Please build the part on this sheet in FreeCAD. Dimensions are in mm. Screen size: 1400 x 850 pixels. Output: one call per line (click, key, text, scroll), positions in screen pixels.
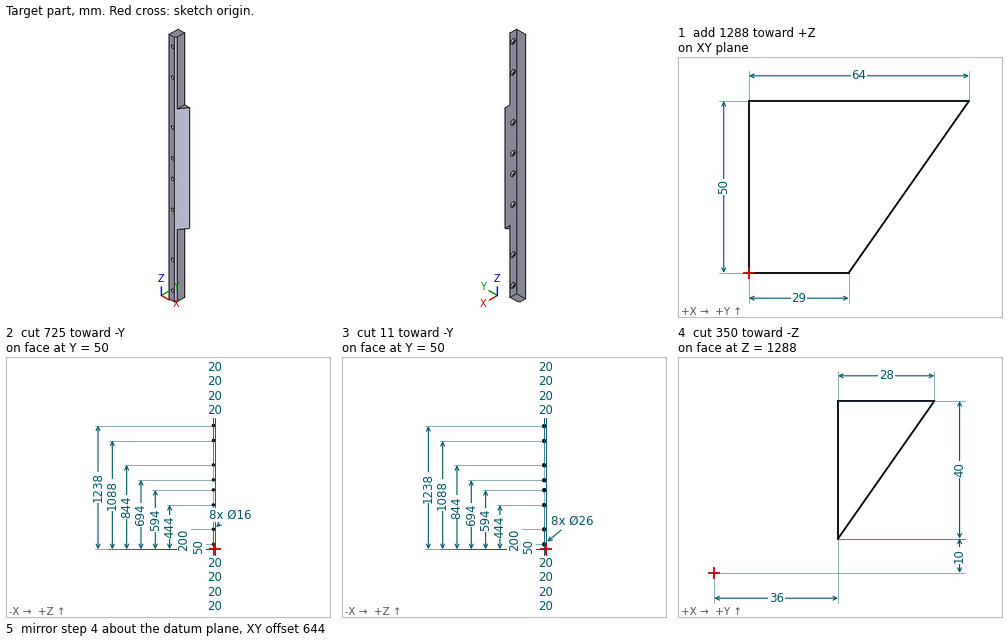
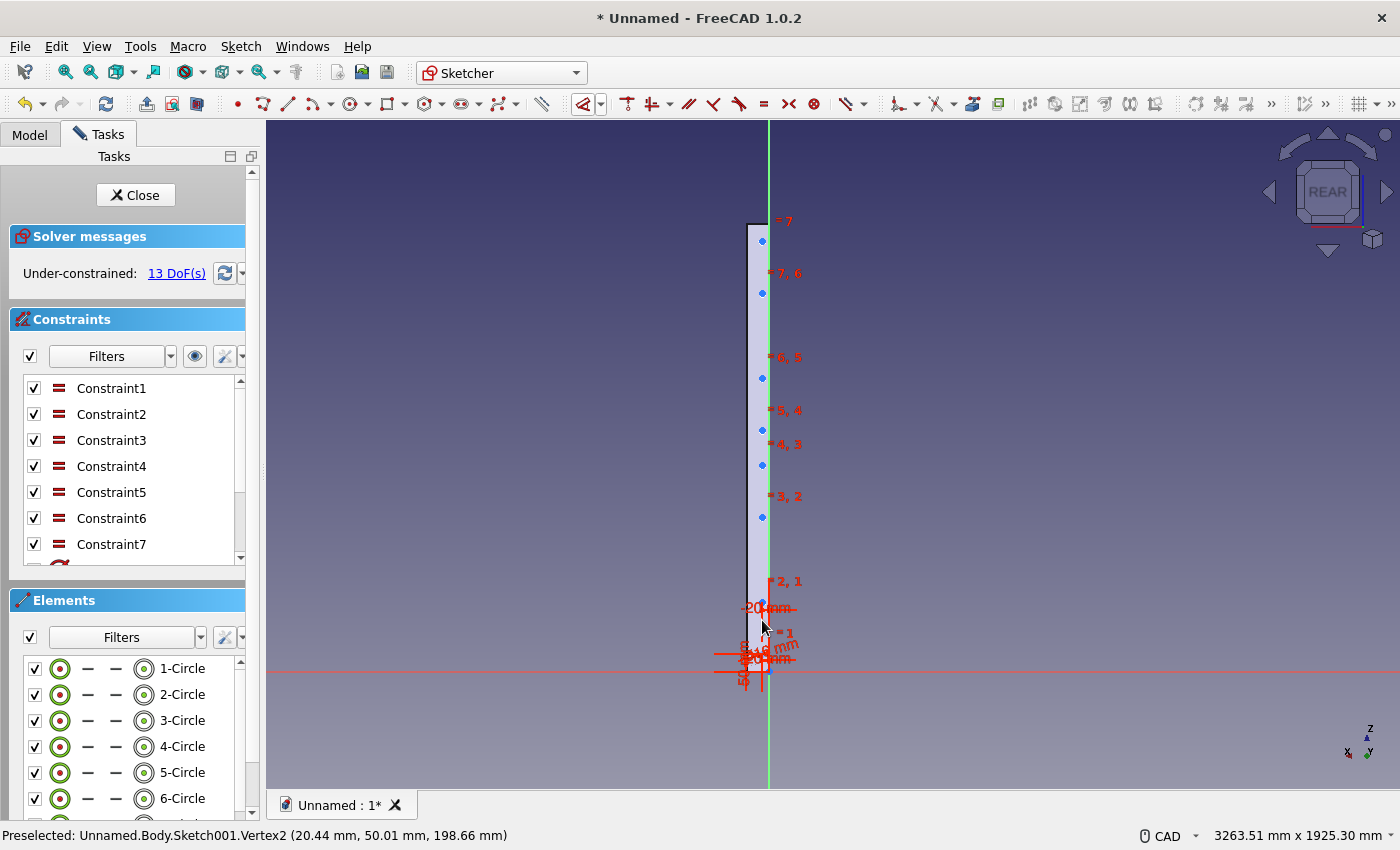
scroll(762, 518, up, 9)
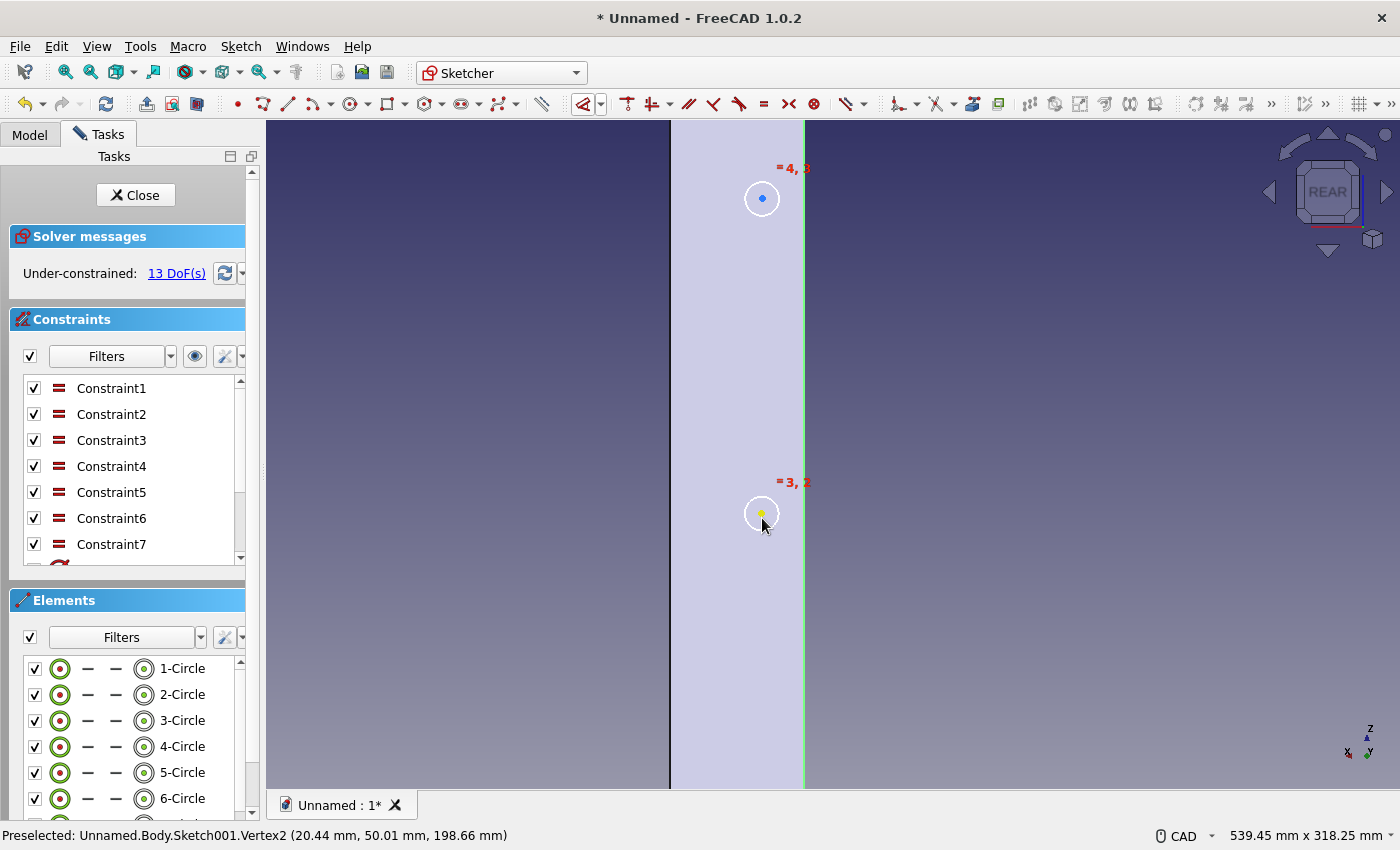
click(762, 514)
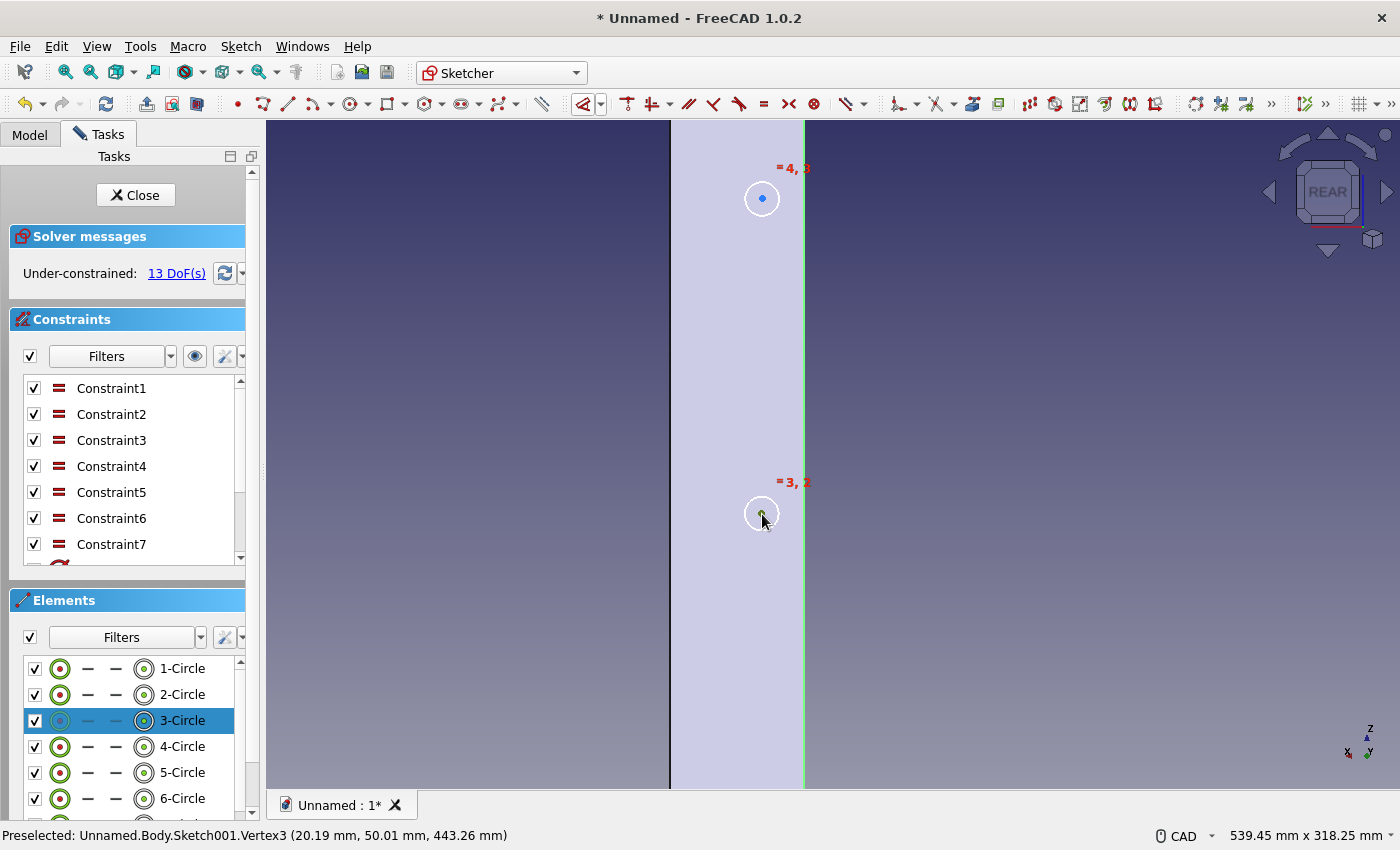
click(600, 104)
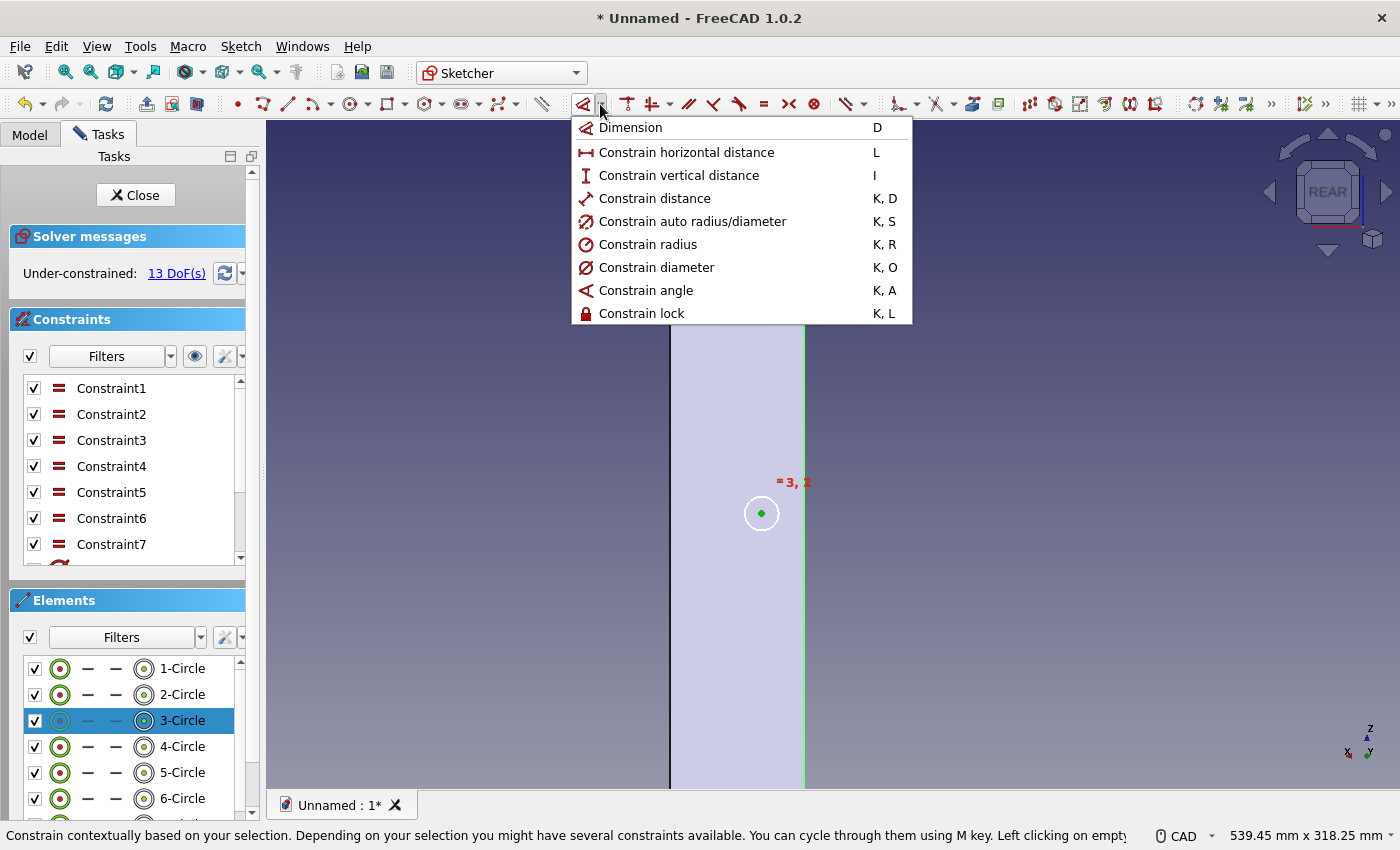
click(742, 152)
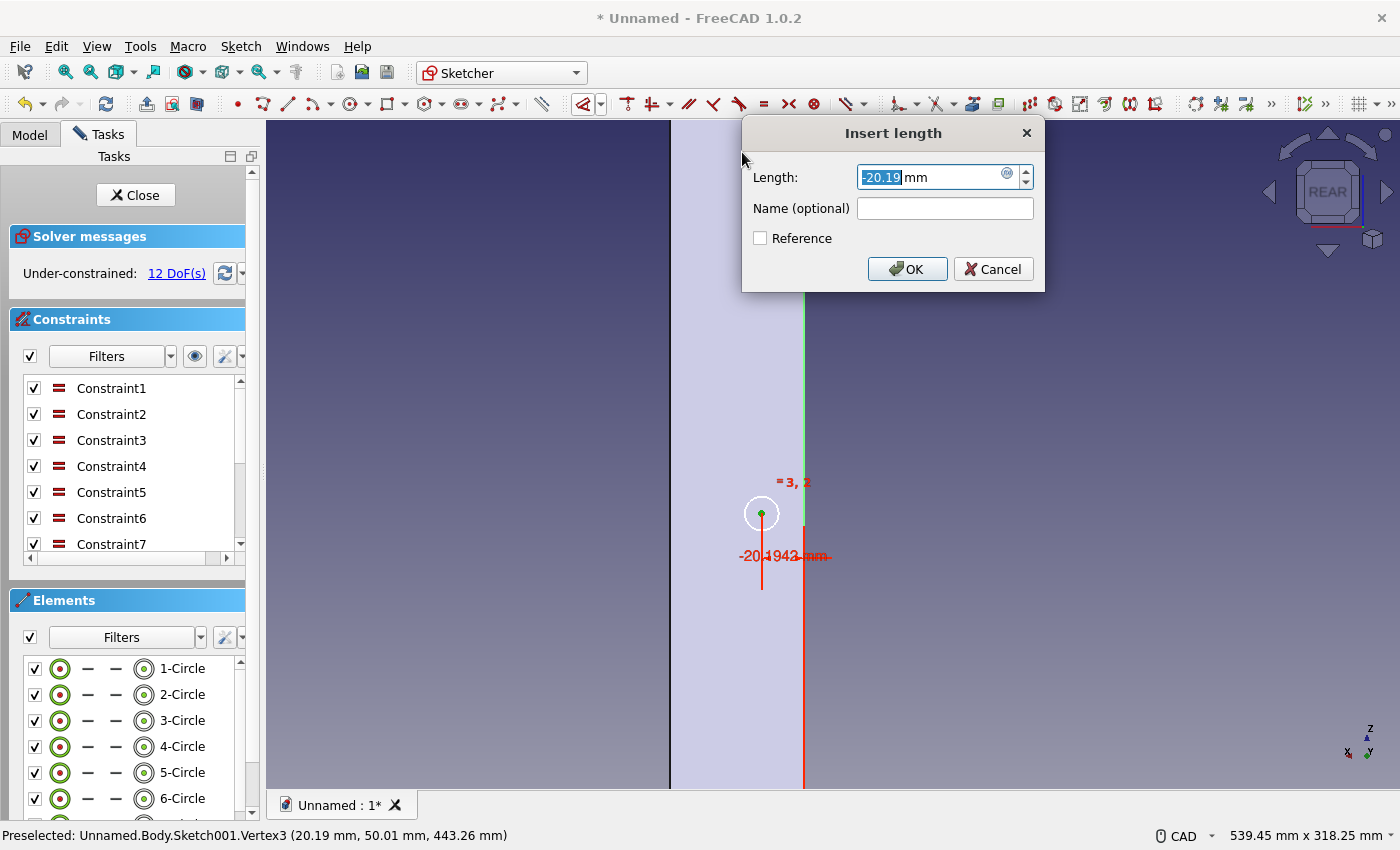
text(-20)
key(Return)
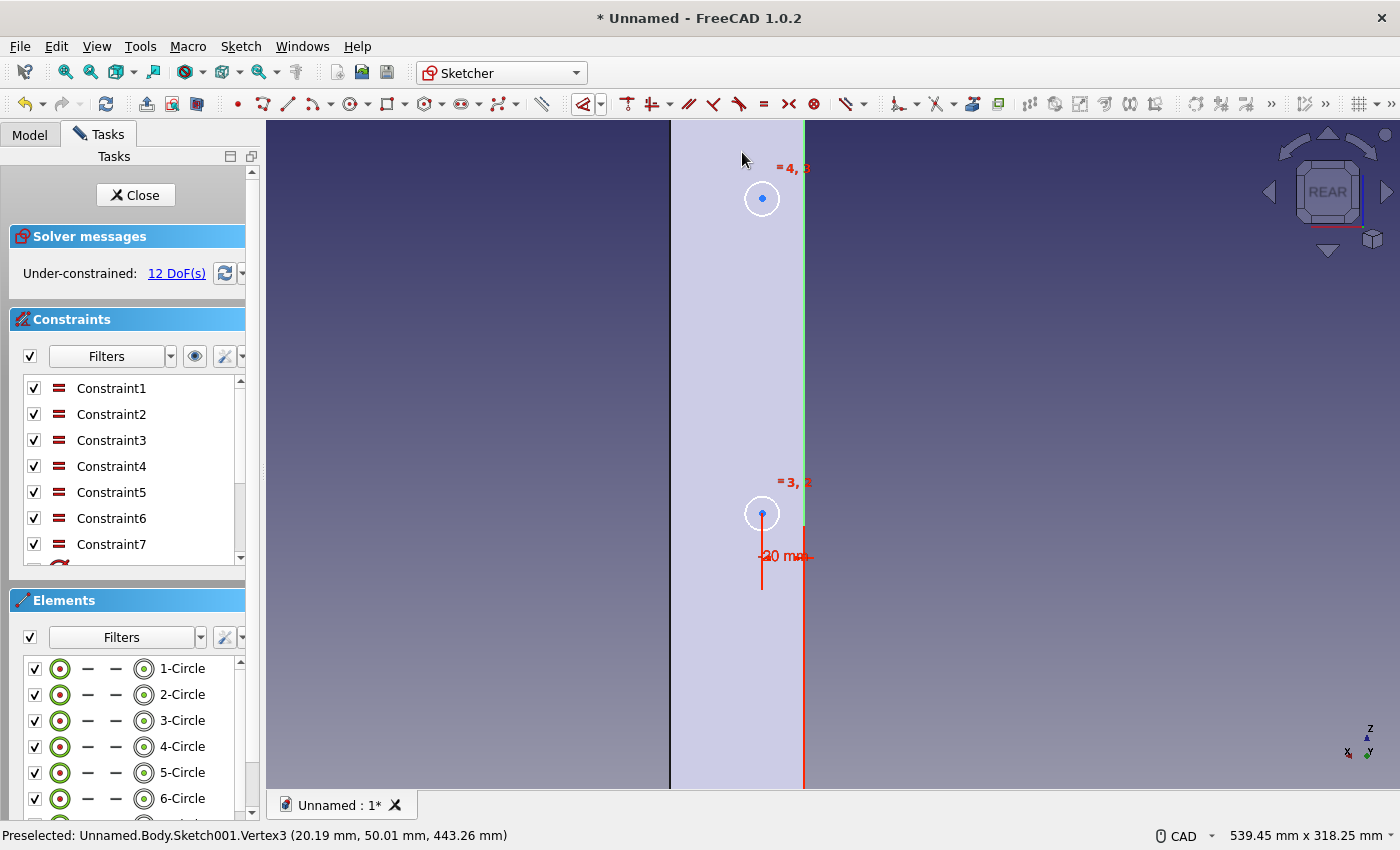
click(762, 199)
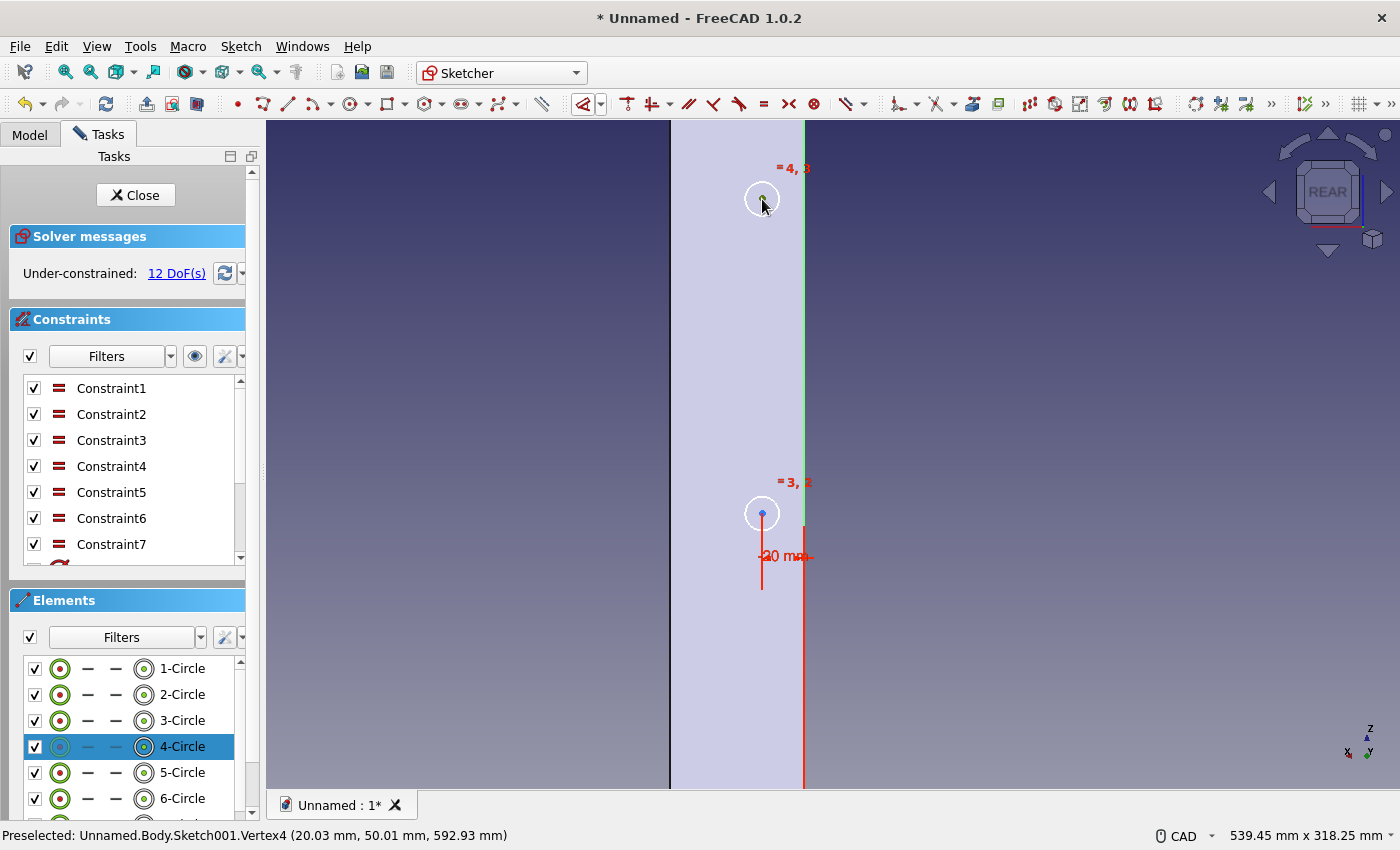
key(l)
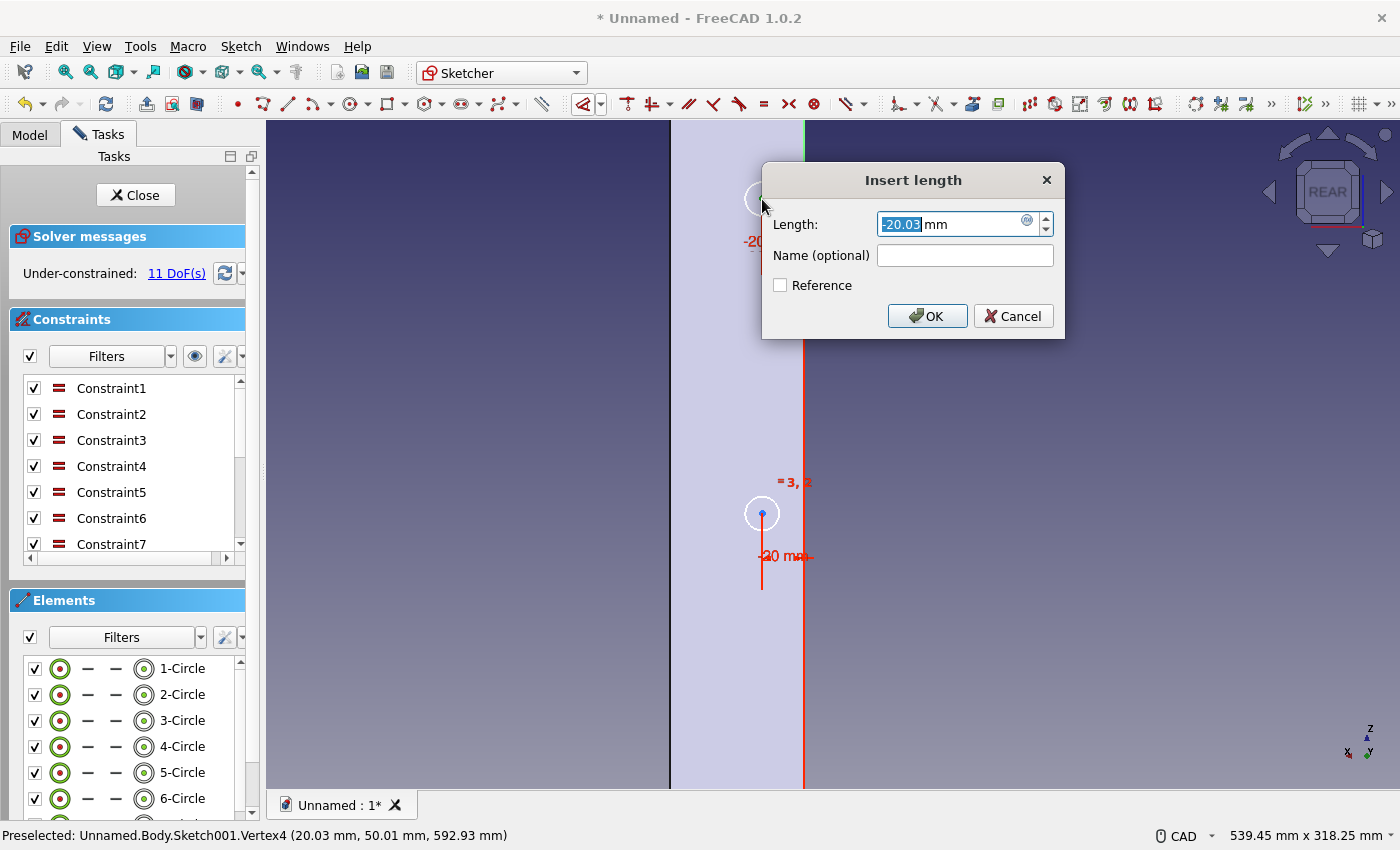
text(-20)
key(Return)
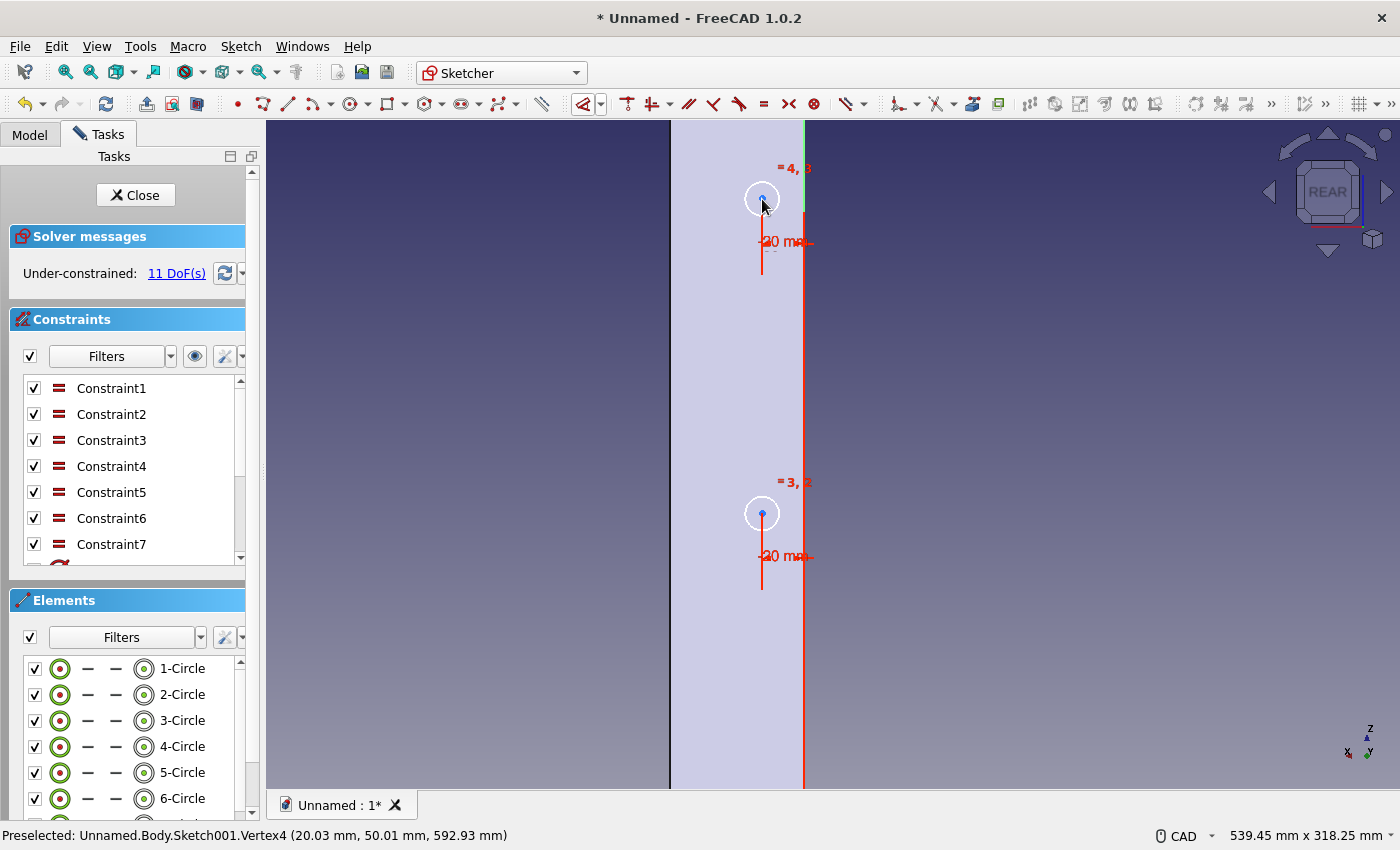
scroll(762, 518, down, 9)